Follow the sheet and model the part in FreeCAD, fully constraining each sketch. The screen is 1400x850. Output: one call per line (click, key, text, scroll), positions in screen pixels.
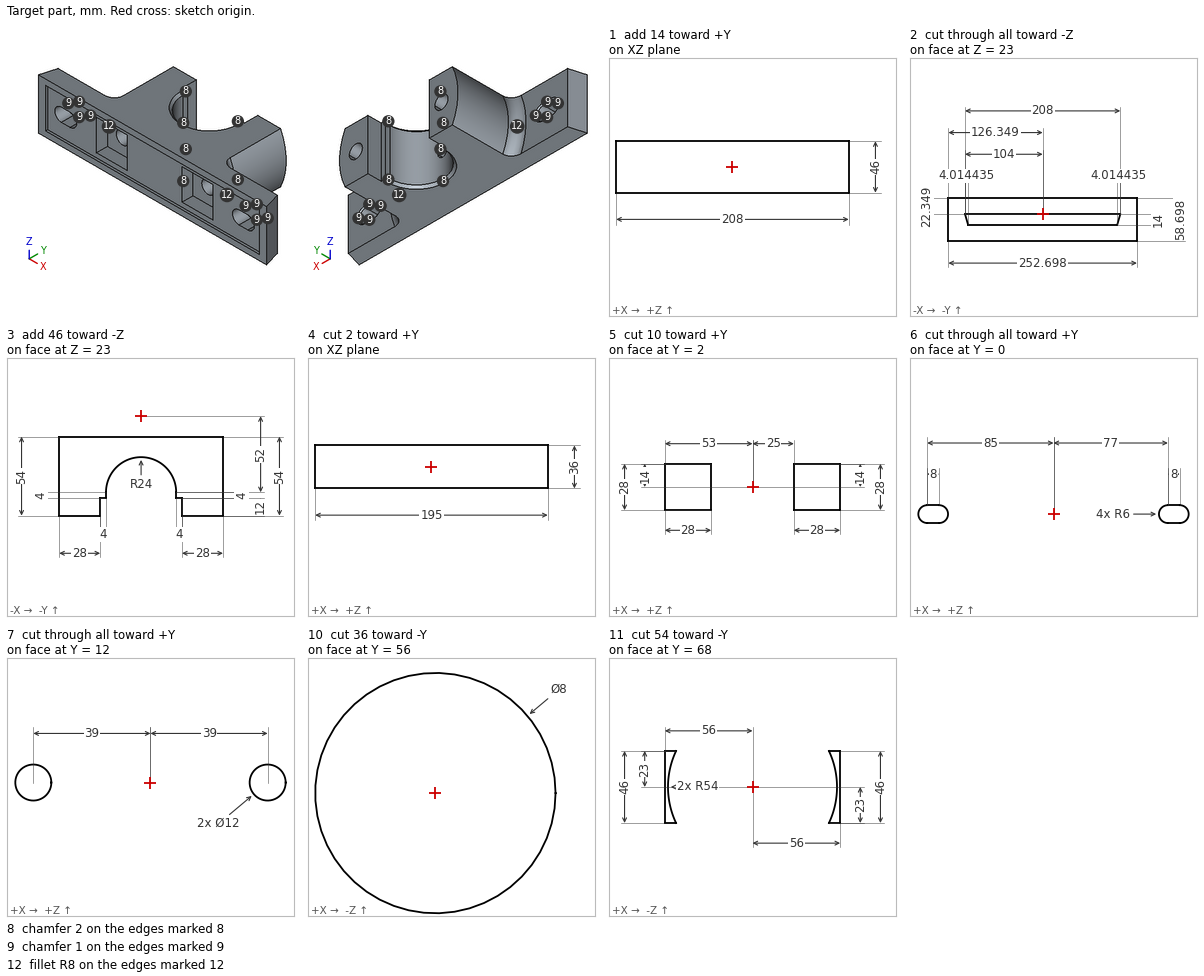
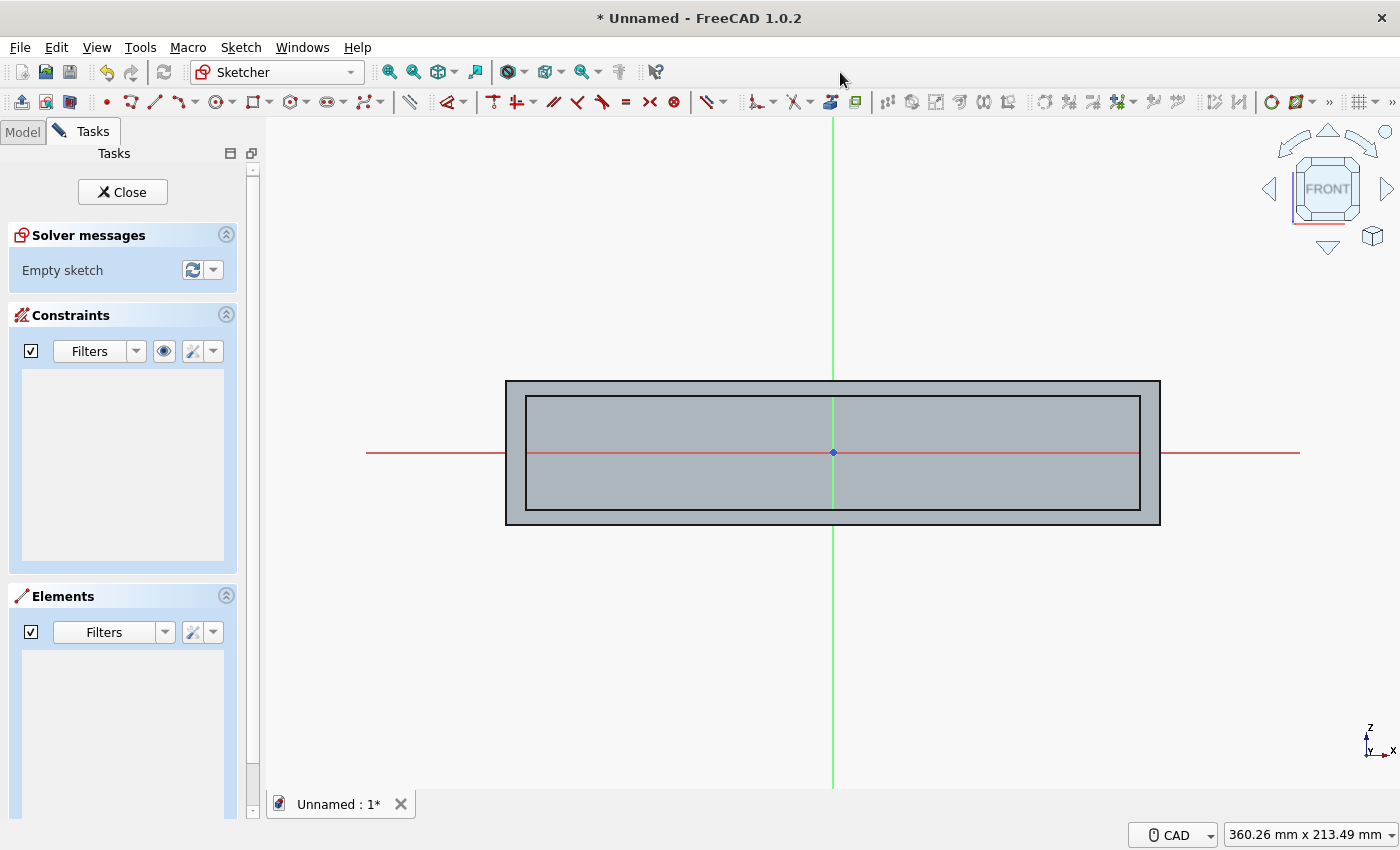
scroll(916, 453, up, 3)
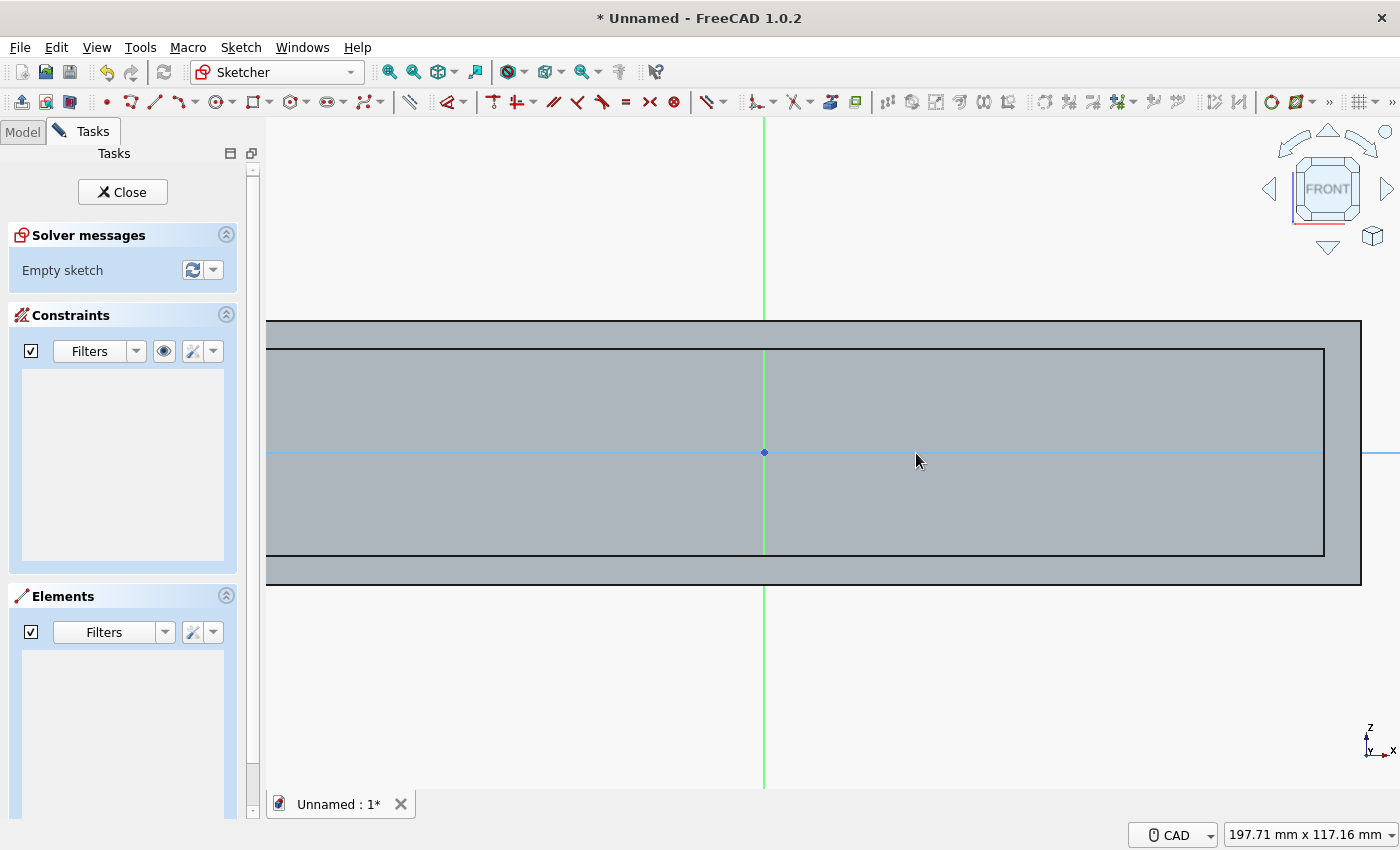
key(g)
key(r)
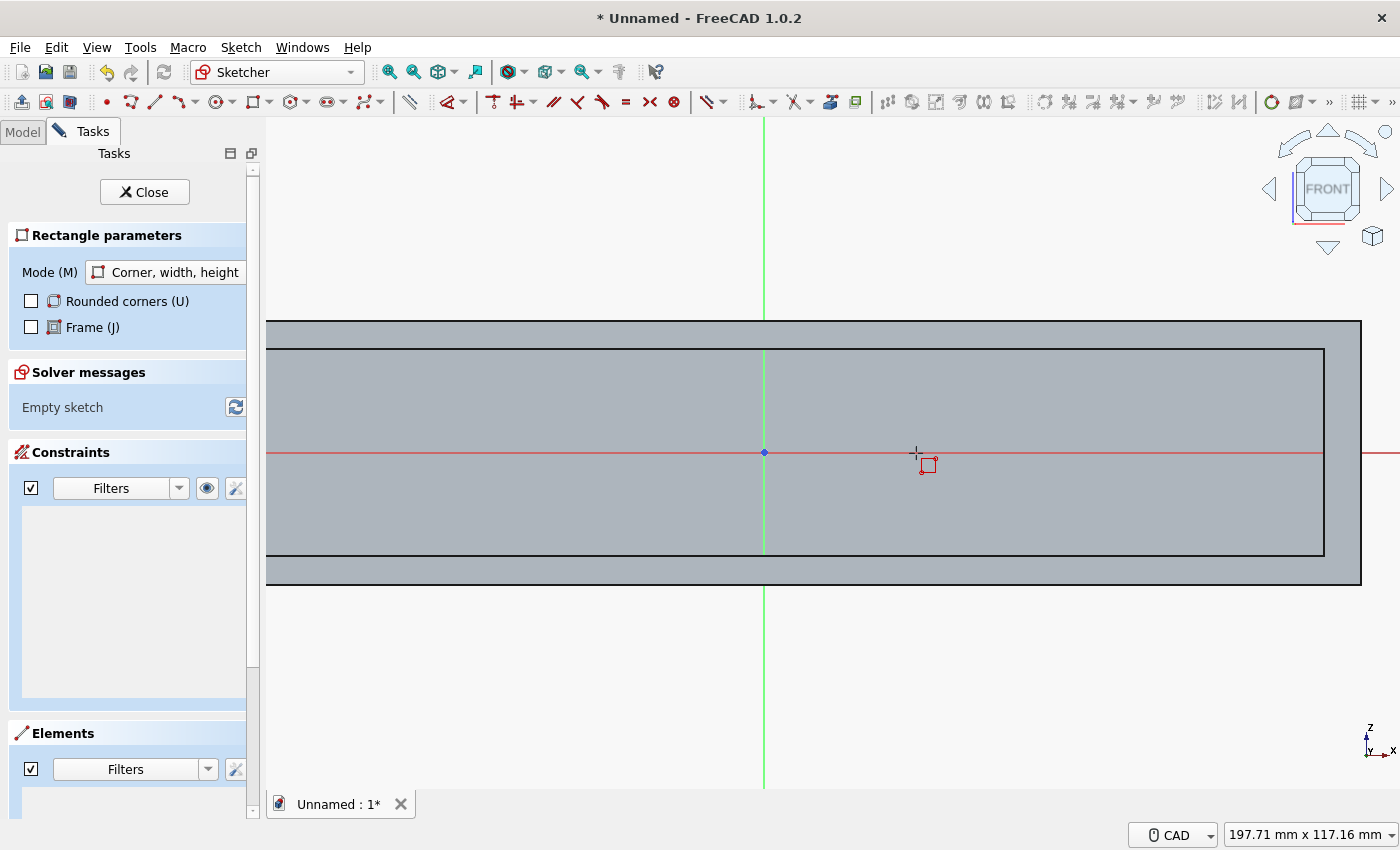
click(908, 372)
move(1068, 533)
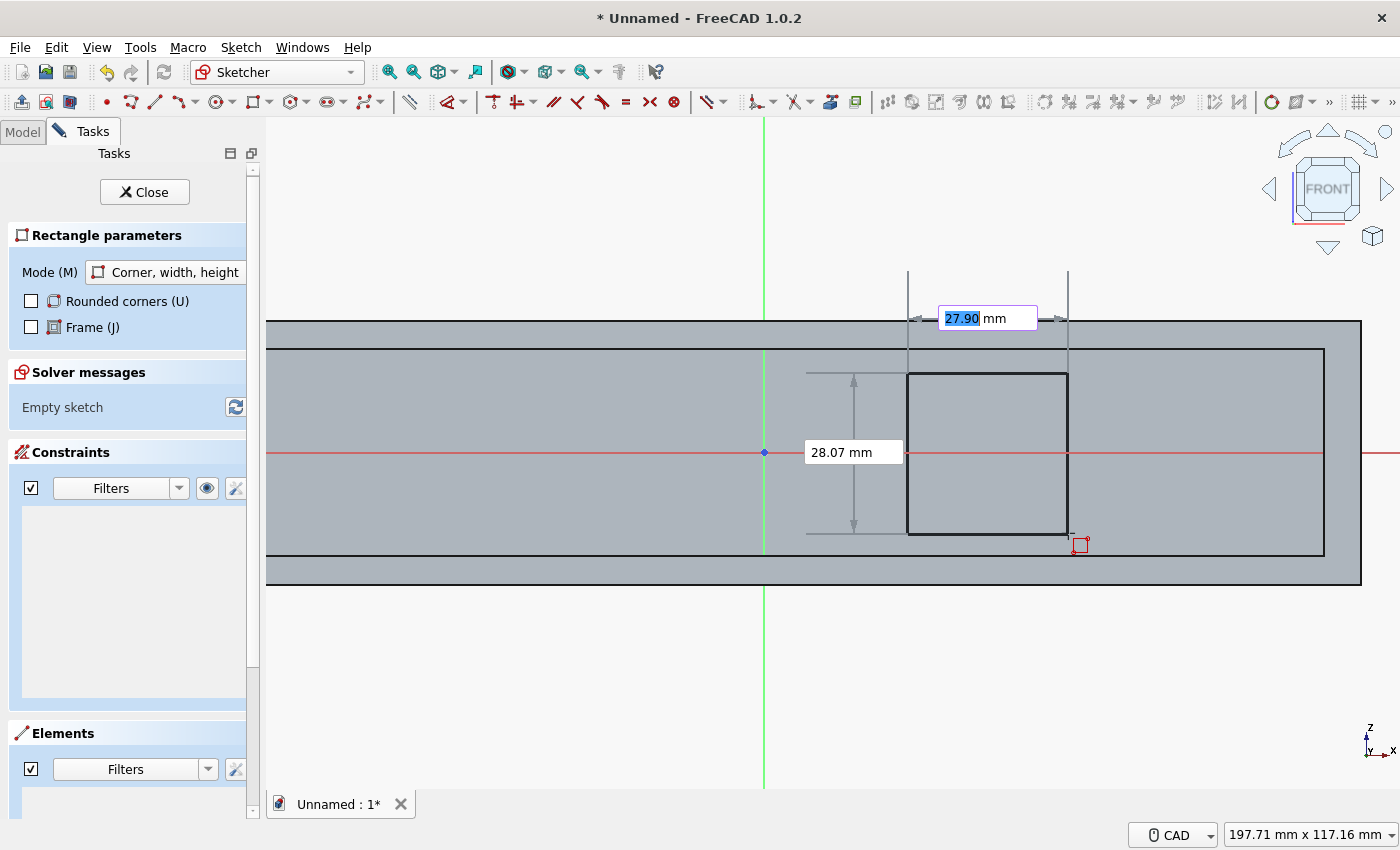
text(28)
key(Tab)
text(28)
key(Return)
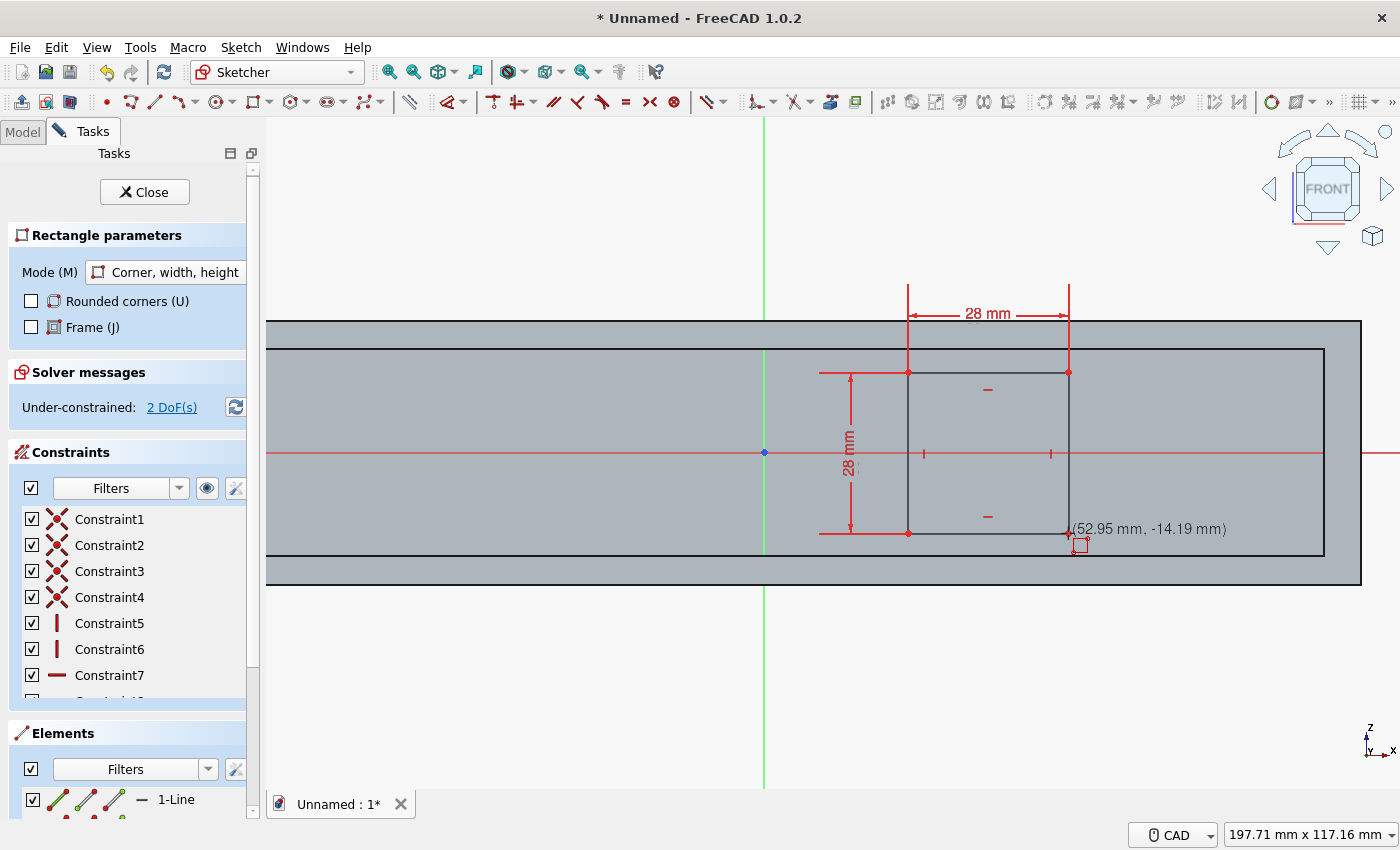
click(460, 372)
move(621, 533)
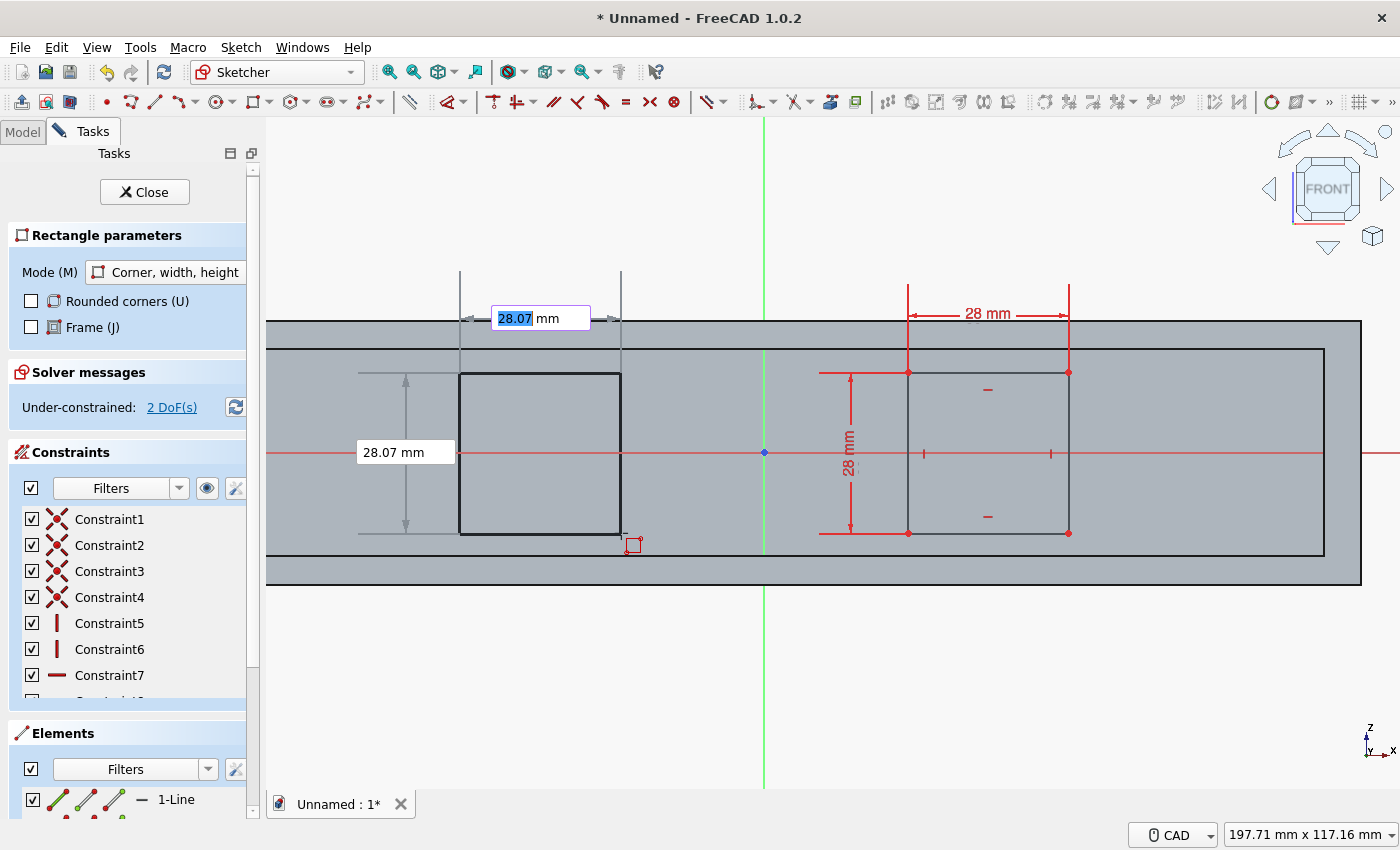
text(28)
key(Tab)
text(28)
key(Return)
key(Escape)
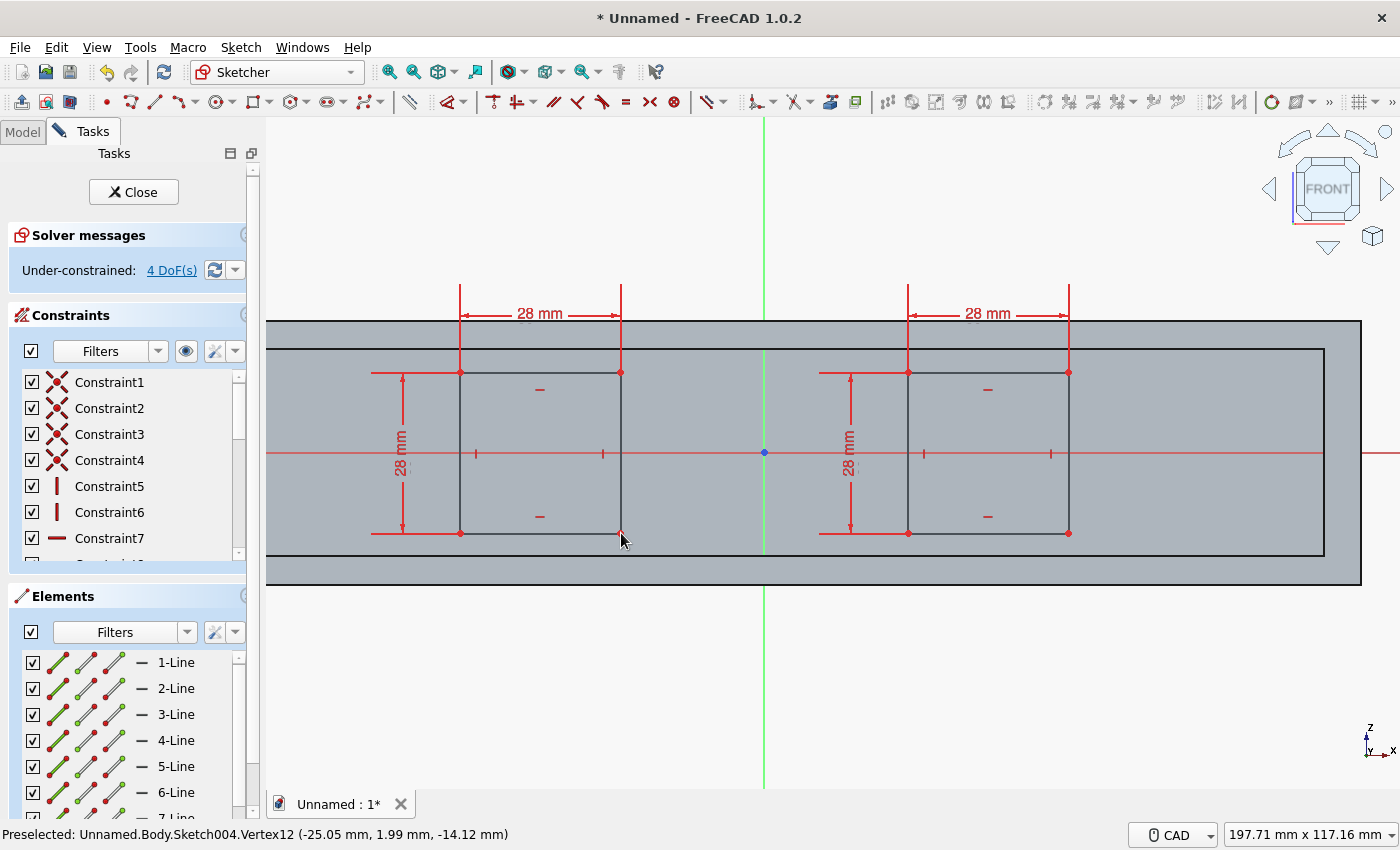
click(448, 102)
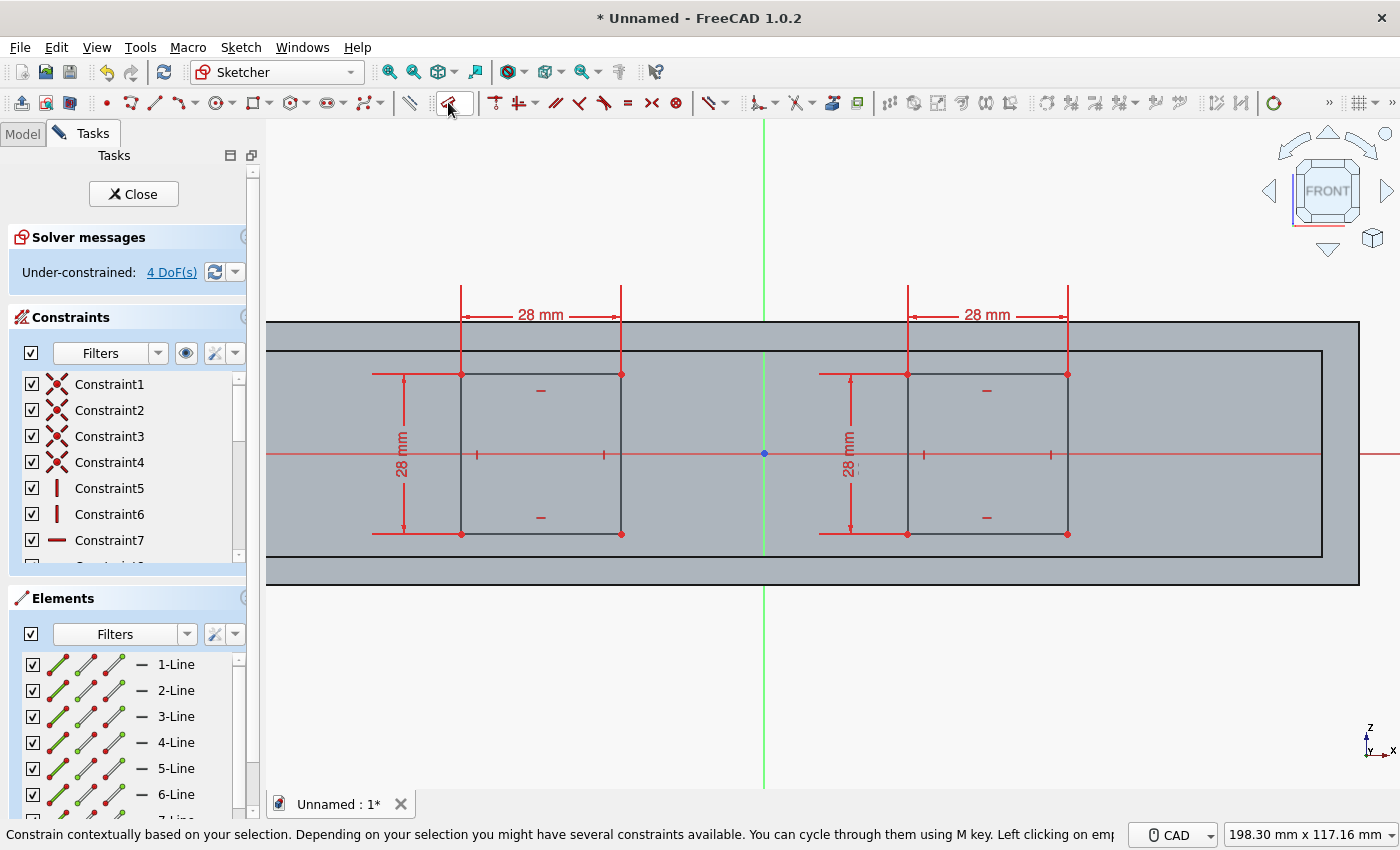
click(908, 374)
click(836, 340)